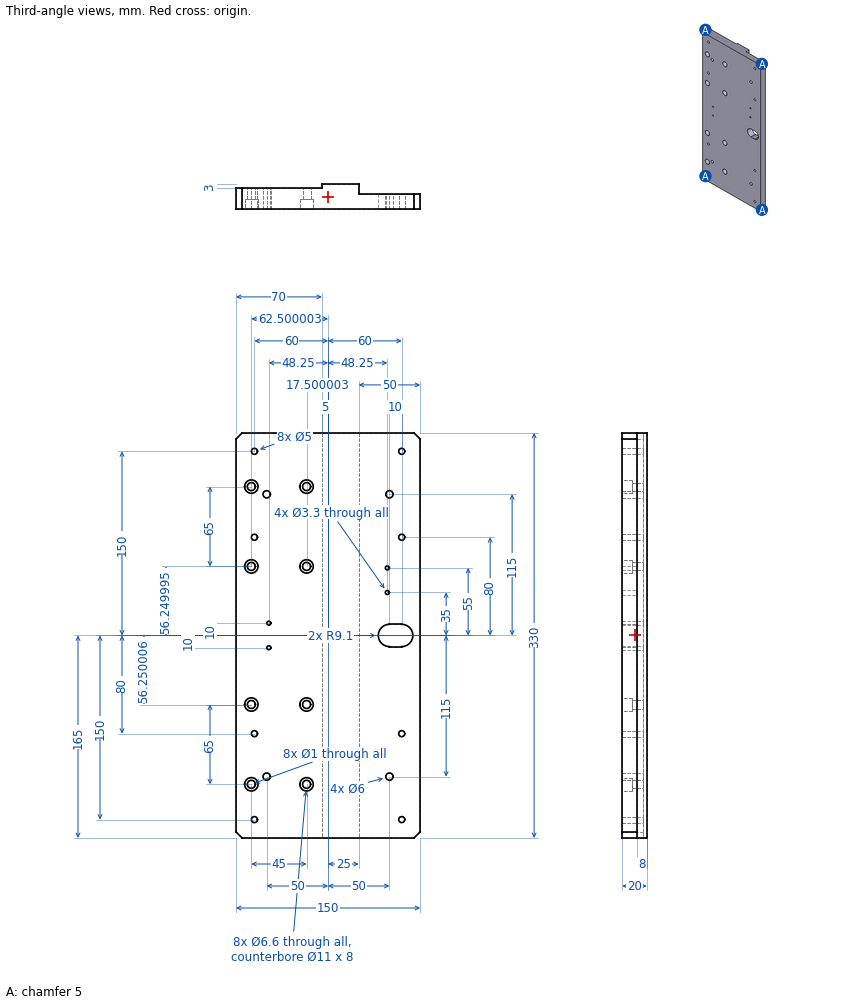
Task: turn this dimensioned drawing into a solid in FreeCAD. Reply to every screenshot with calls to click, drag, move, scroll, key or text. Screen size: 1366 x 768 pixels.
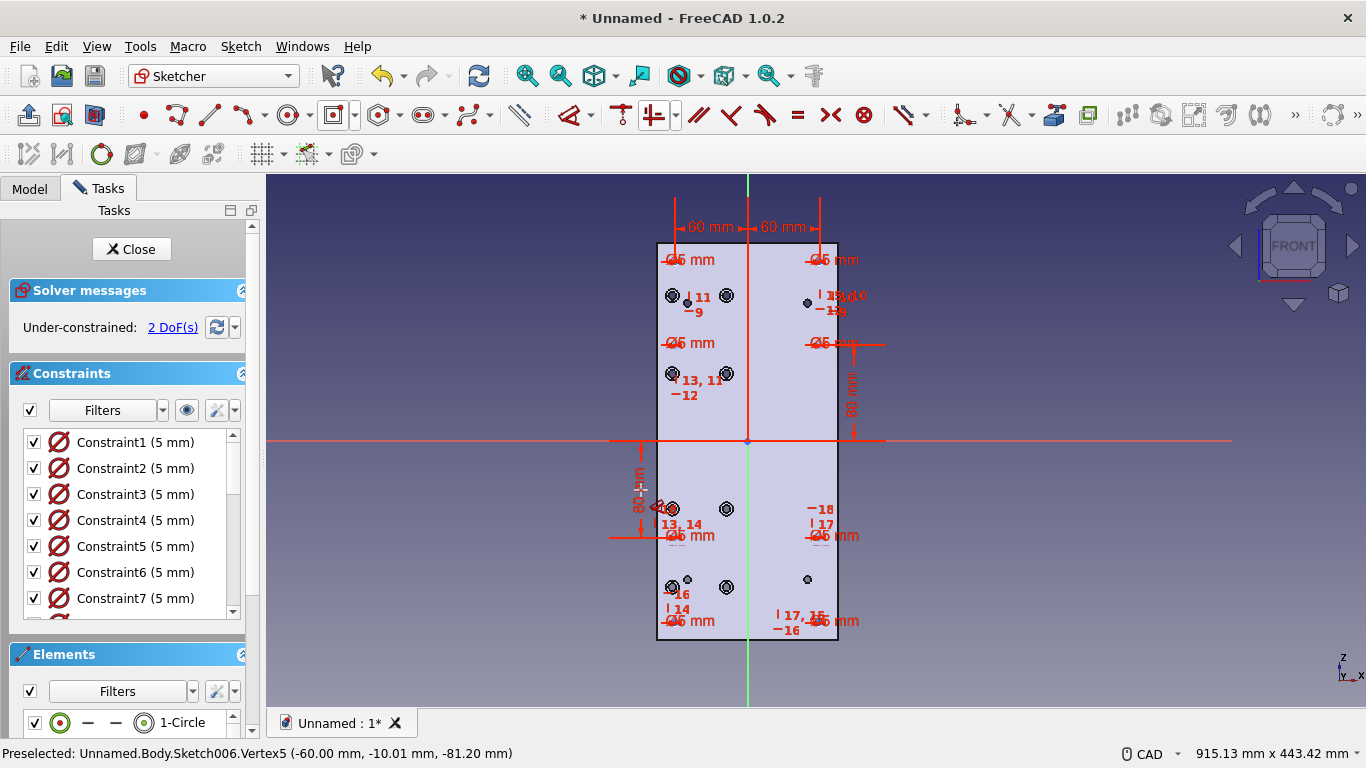
click(675, 262)
click(641, 352)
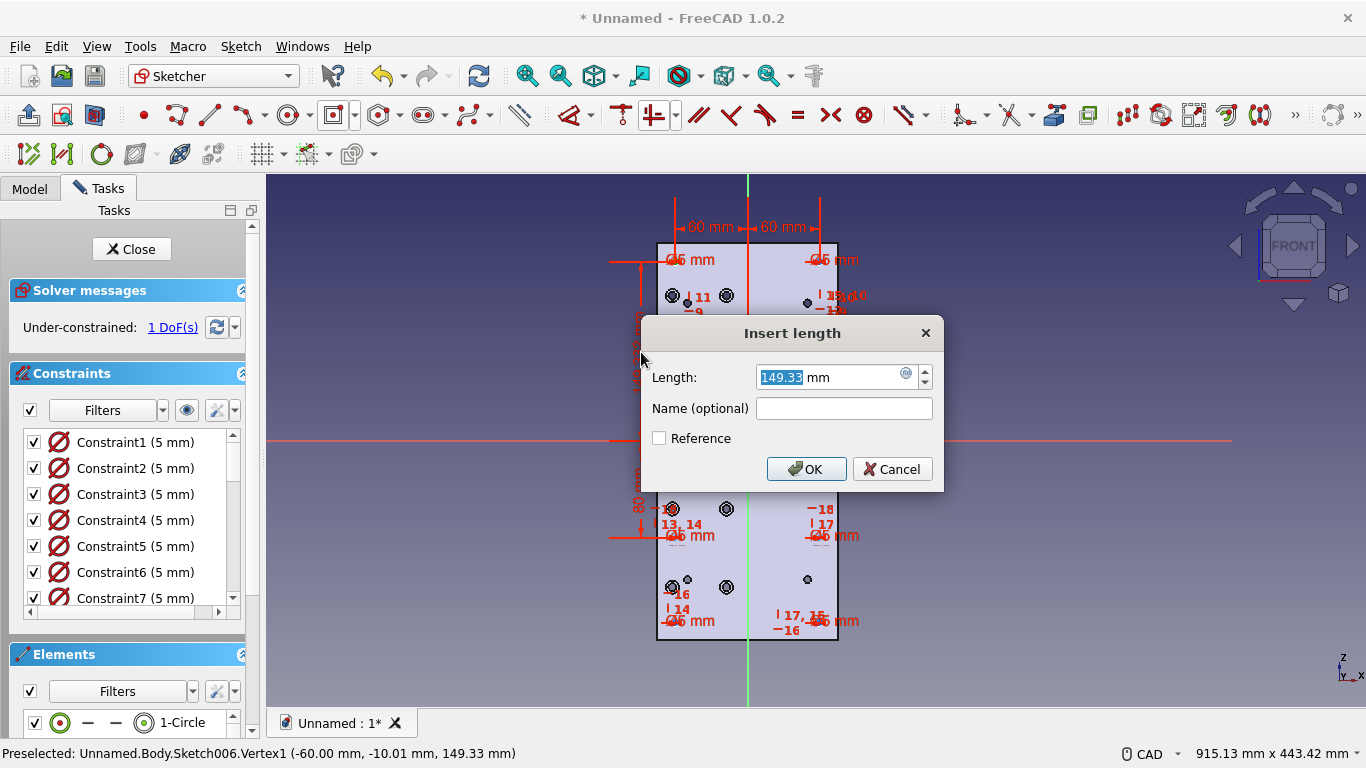
text(150)
key(Return)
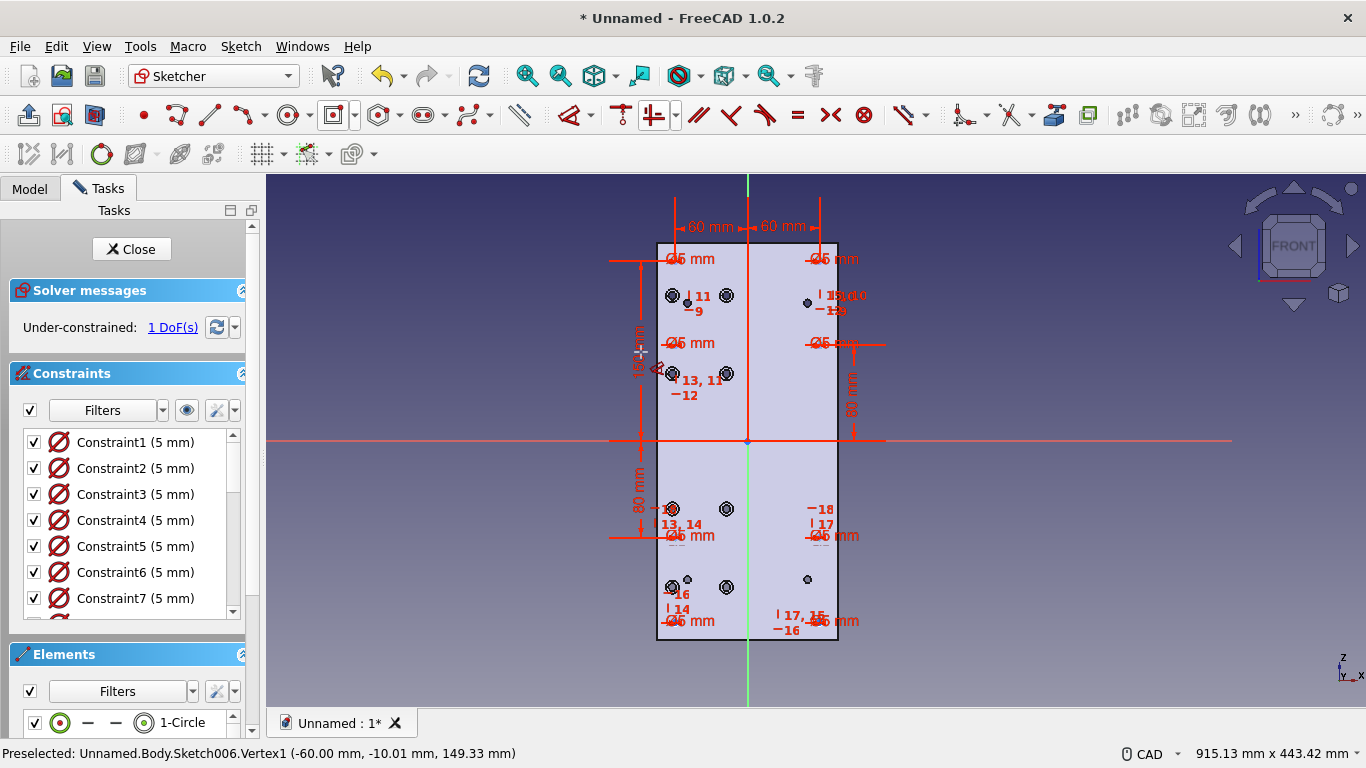
click(675, 623)
click(641, 532)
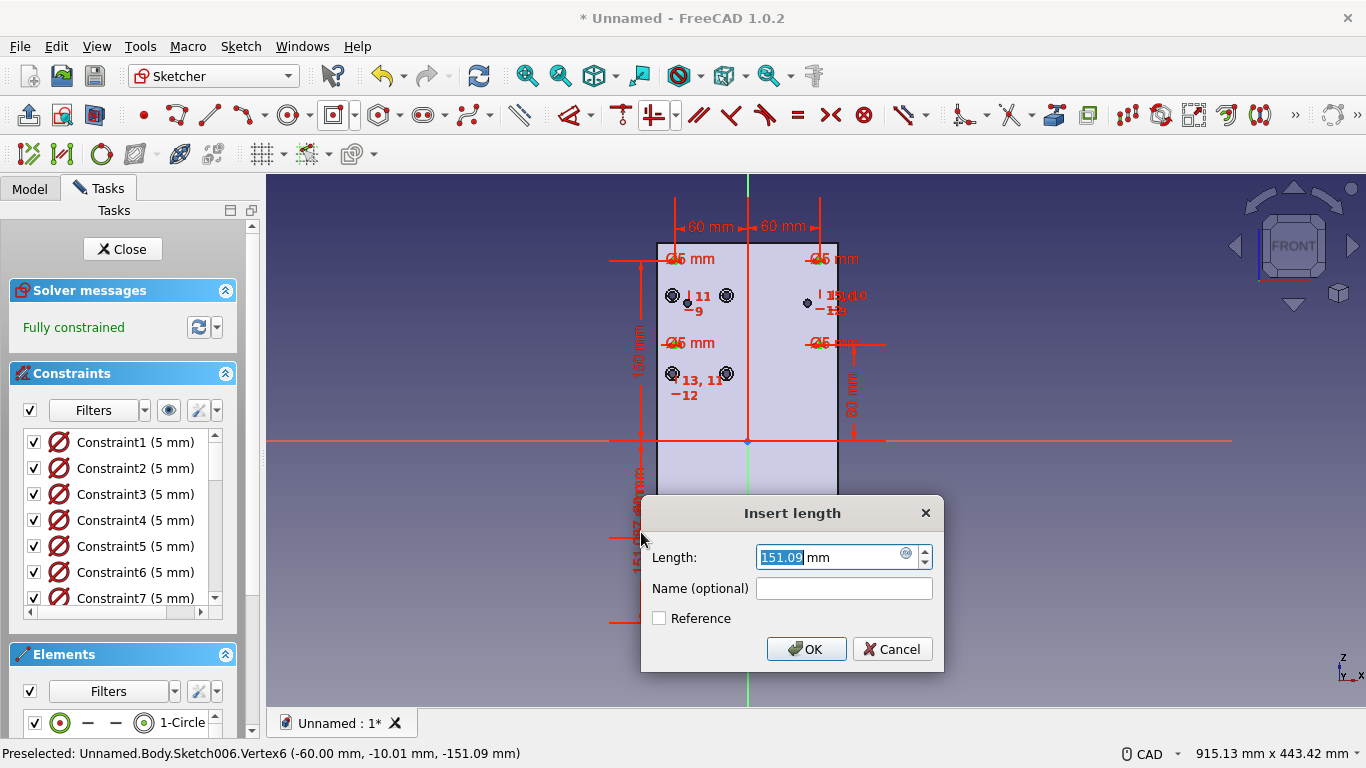
text(150)
key(Return)
key(Escape)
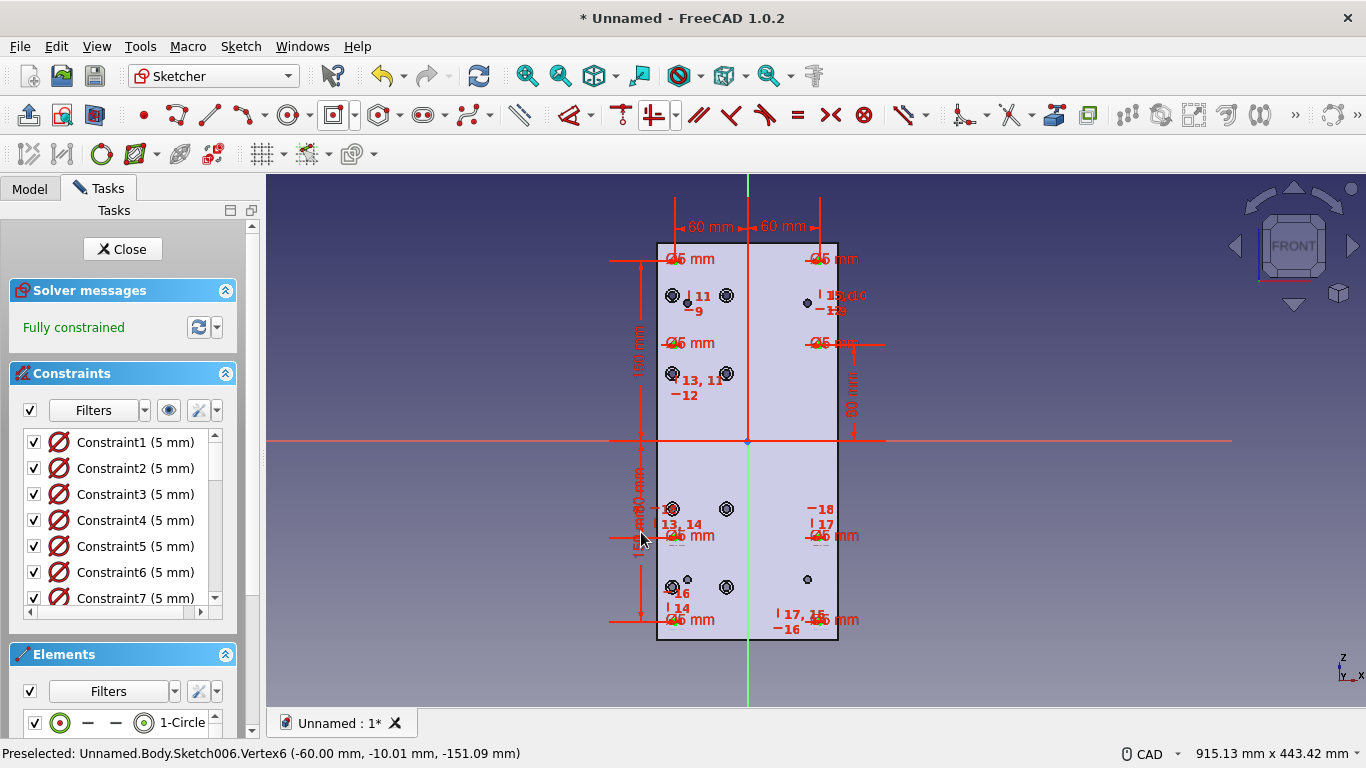
click(123, 249)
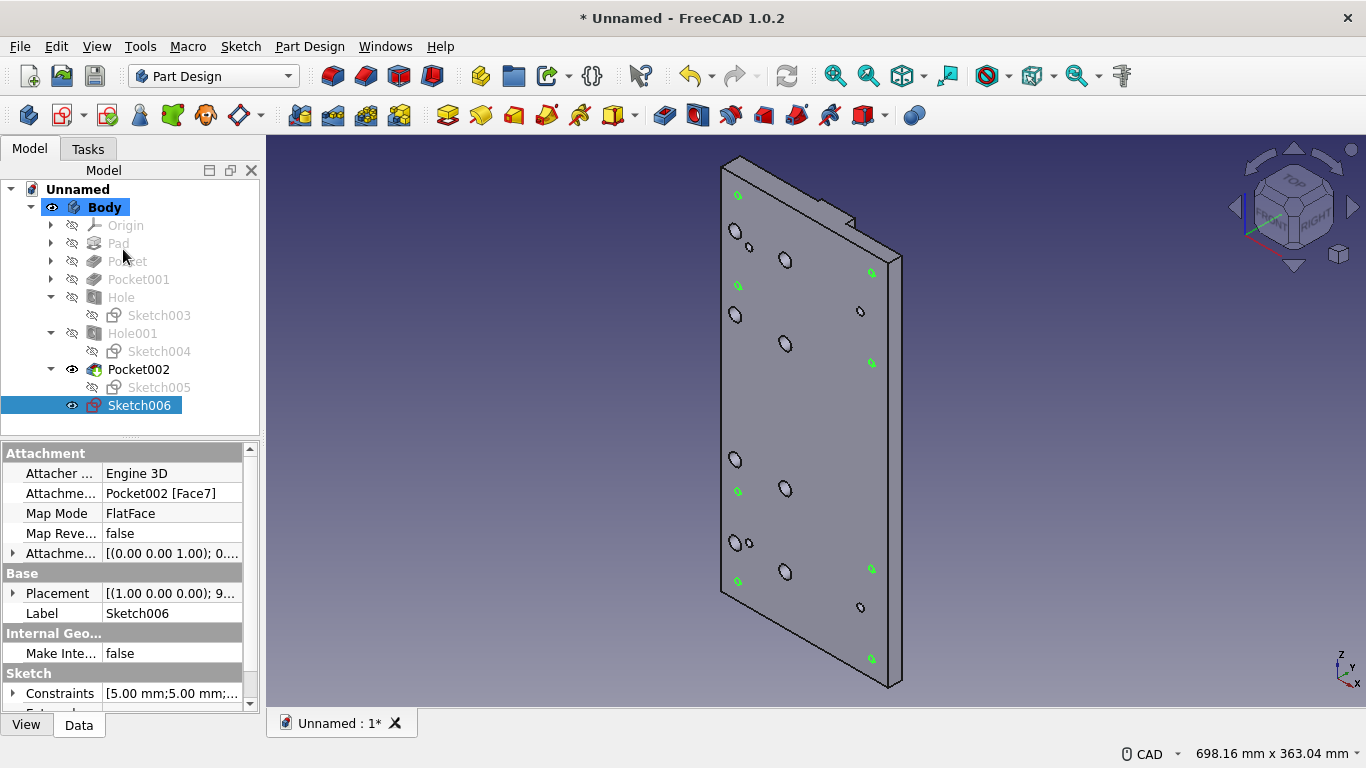
click(665, 116)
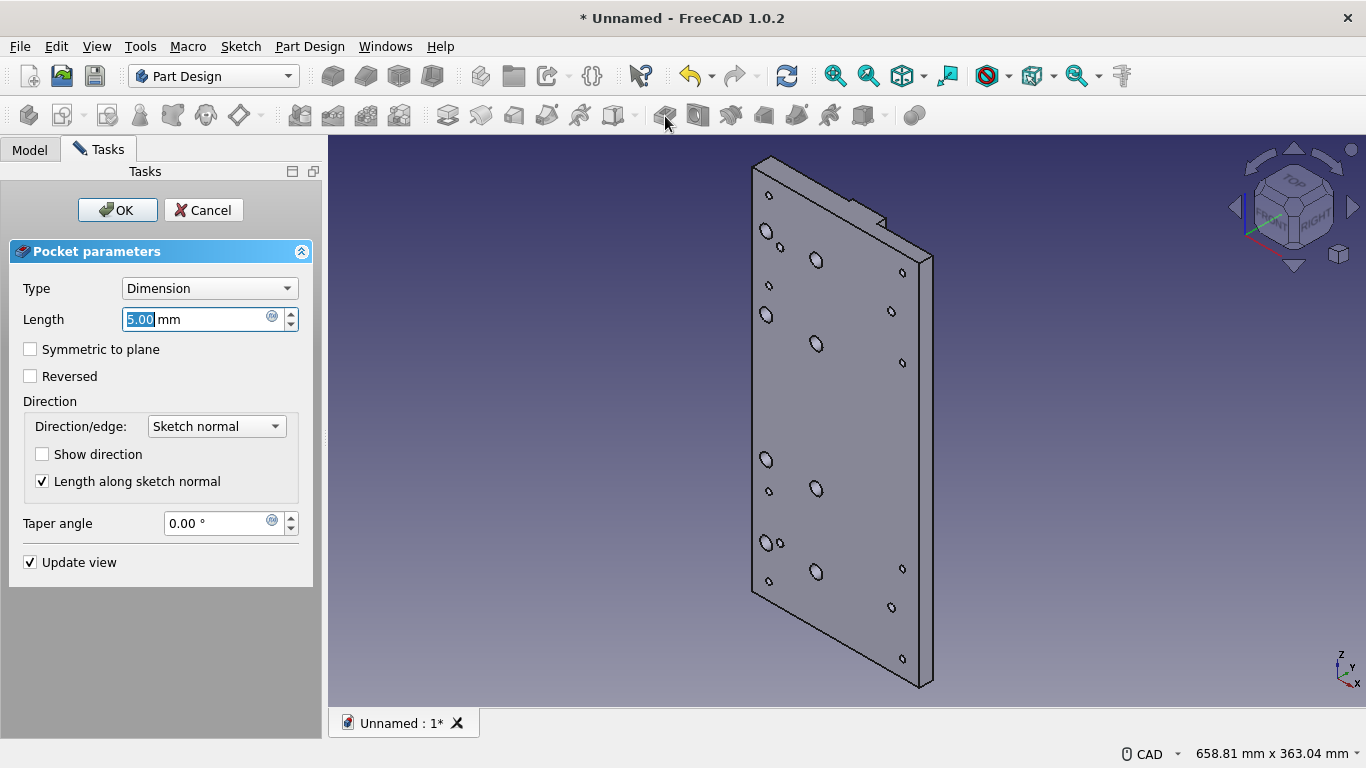
click(210, 288)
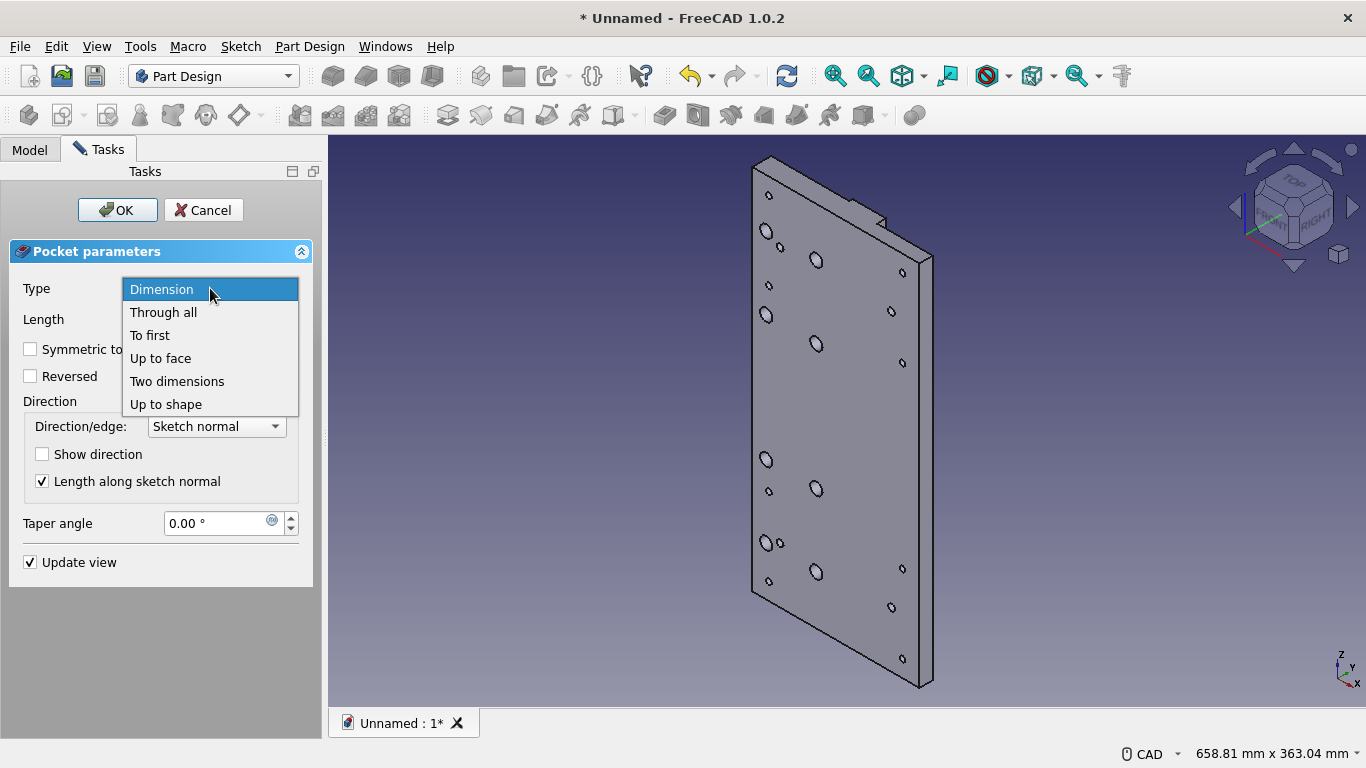
click(208, 312)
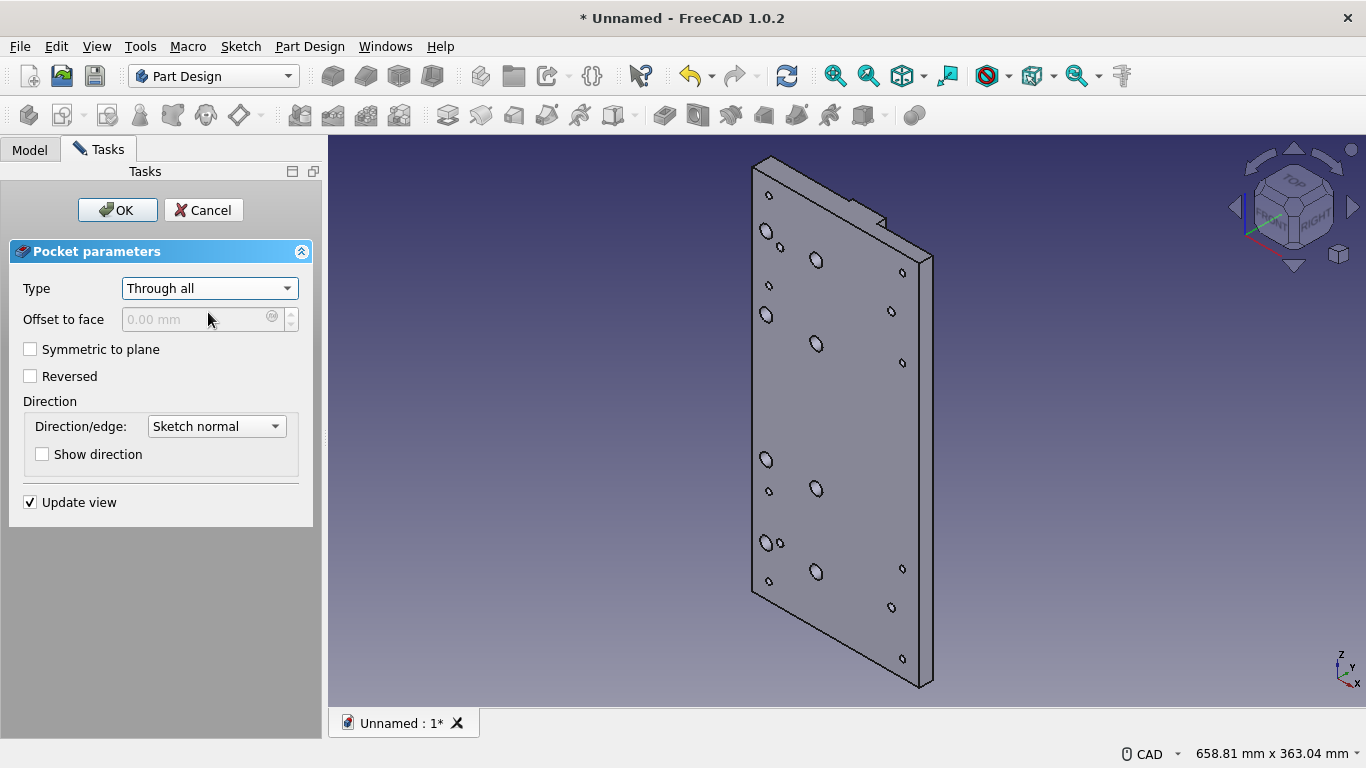
click(118, 210)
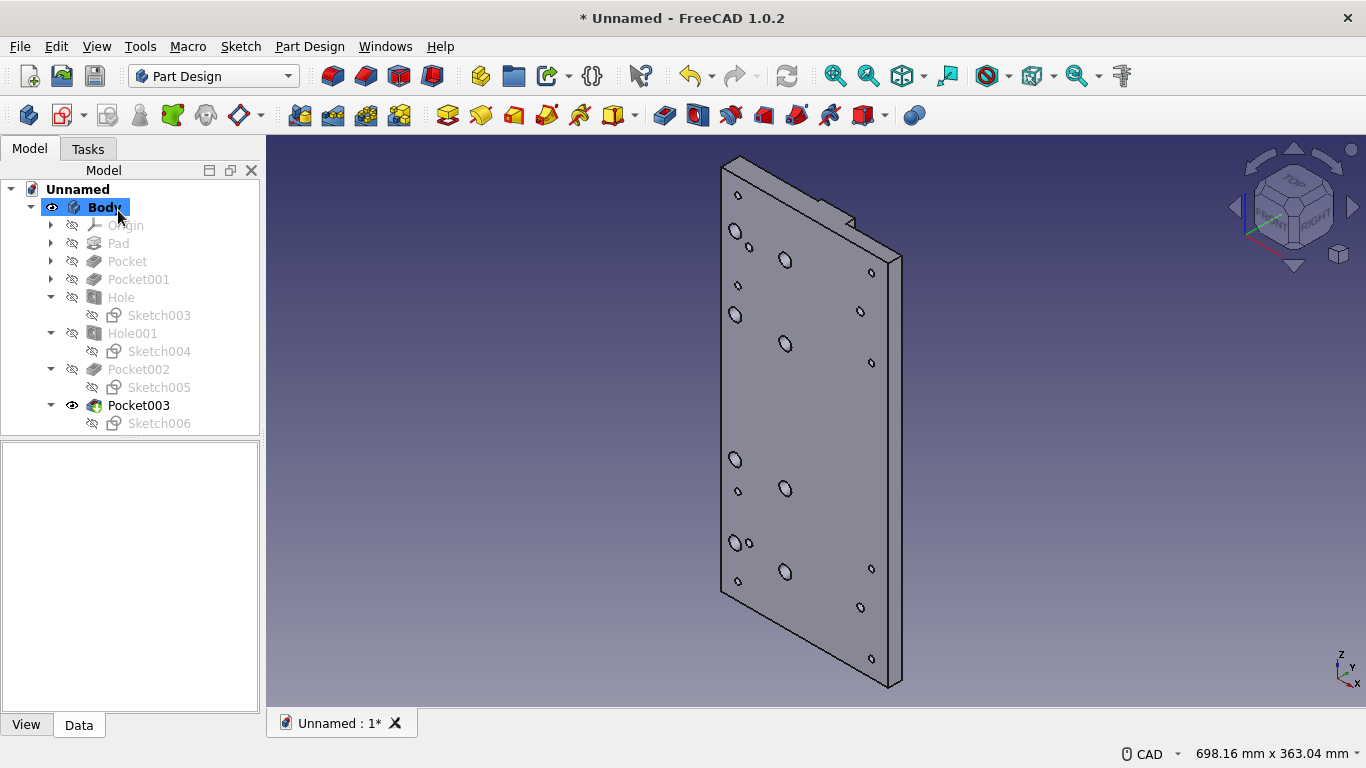
click(895, 259)